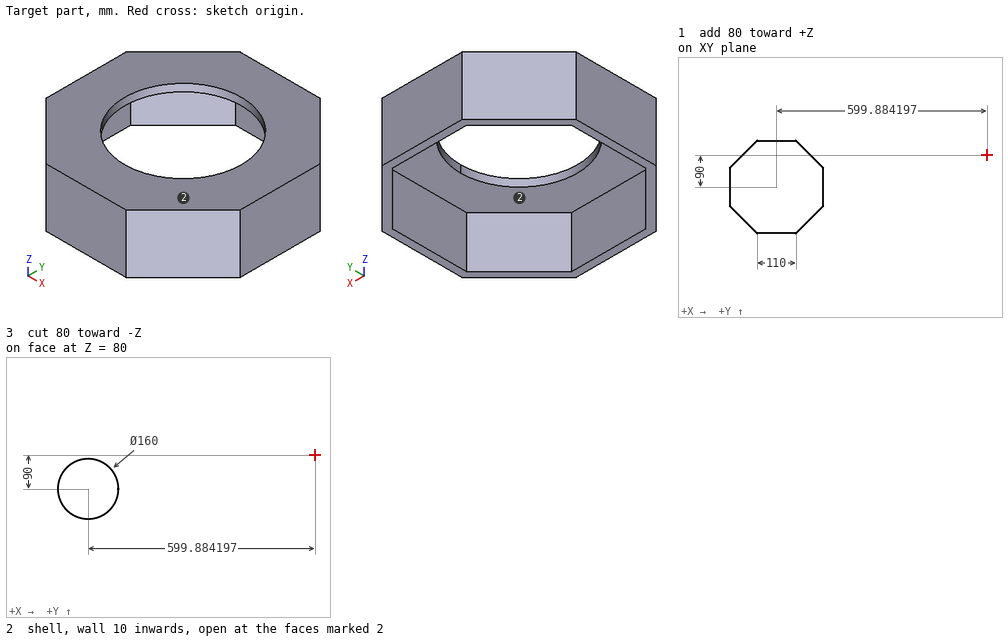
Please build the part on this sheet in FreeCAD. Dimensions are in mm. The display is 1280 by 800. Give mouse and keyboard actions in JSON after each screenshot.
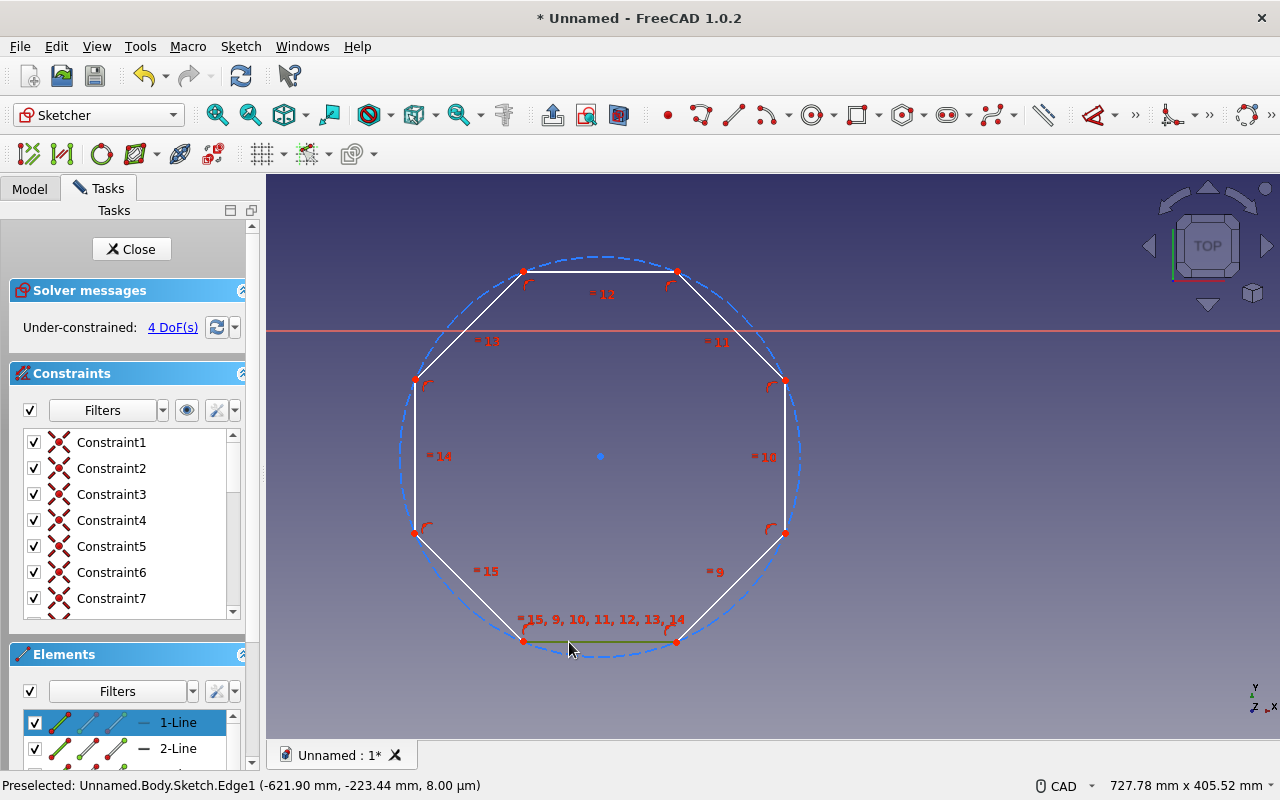
{"action": "key", "text": "h"}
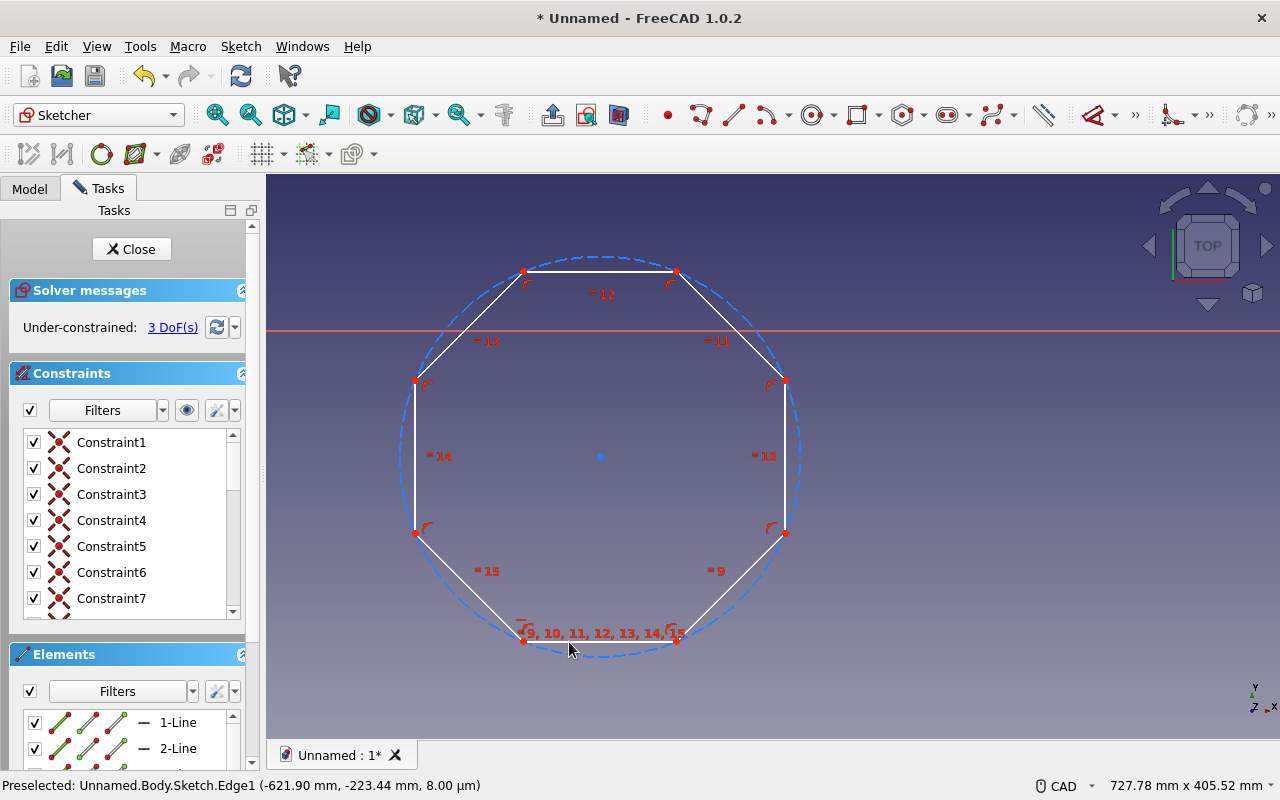
{"action": "left_click", "coordinate": [600, 457]}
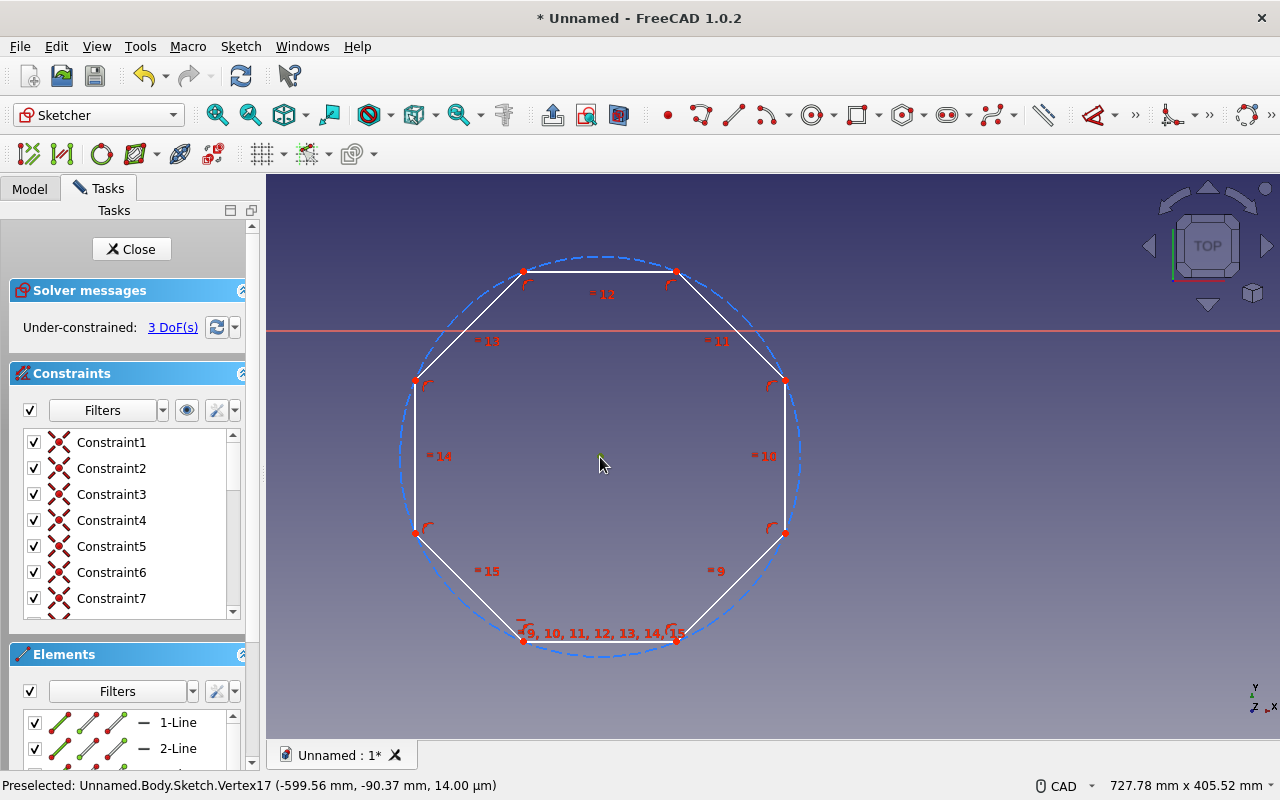
{"action": "key", "text": "i"}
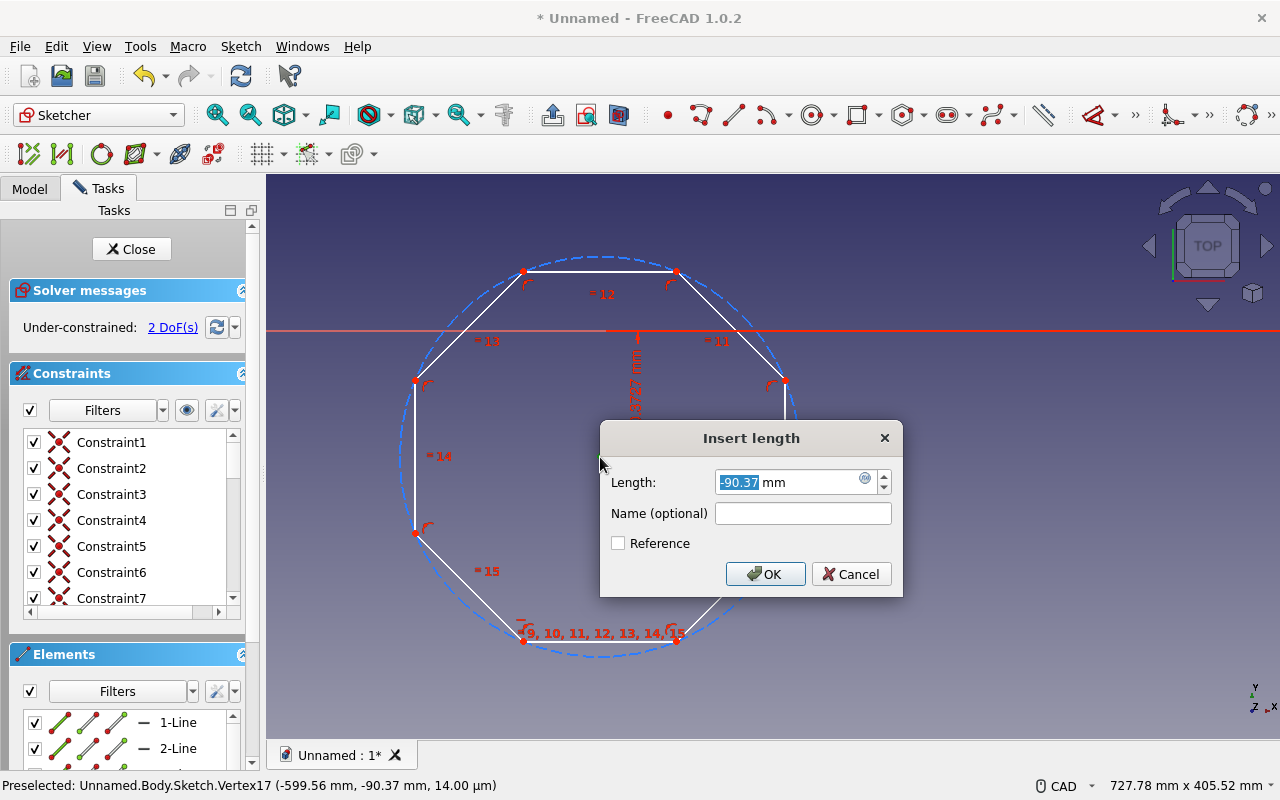
{"action": "type", "text": "-90"}
{"action": "key", "text": "Return"}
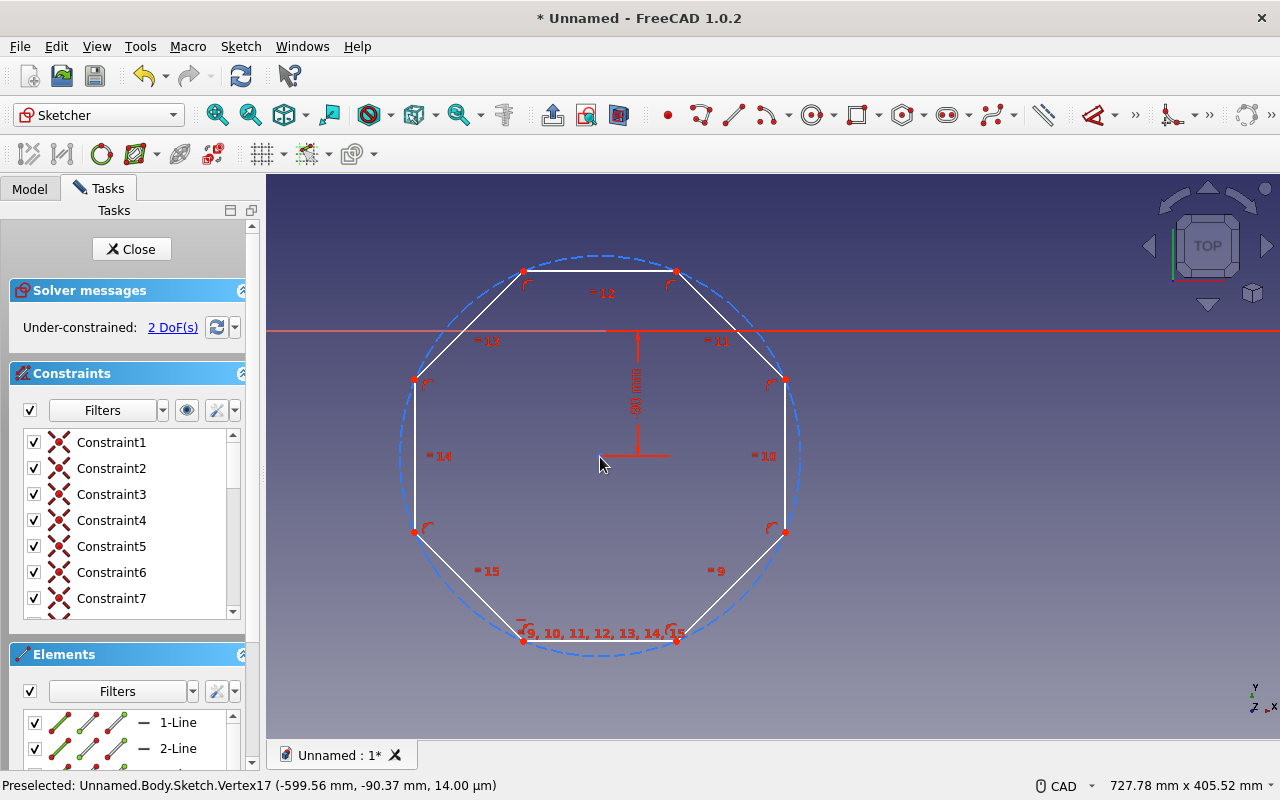
{"action": "left_click", "coordinate": [569, 641]}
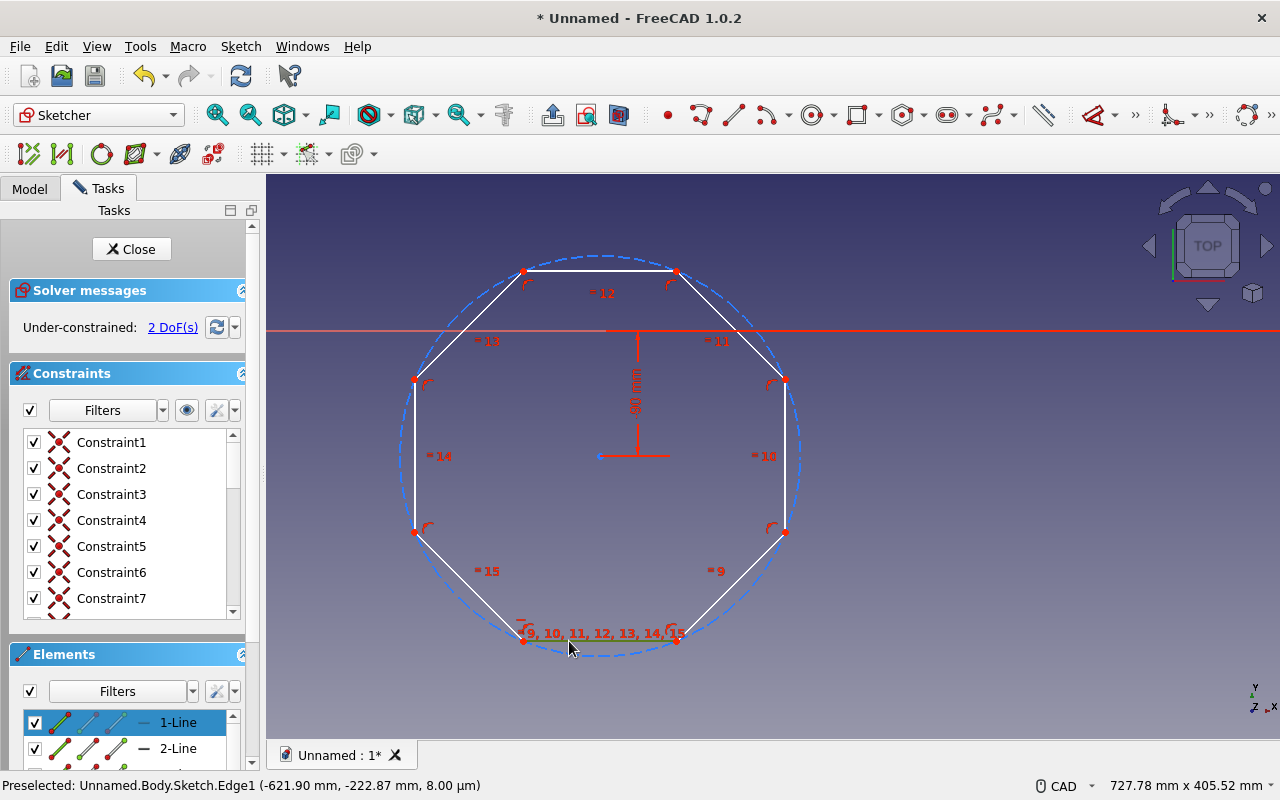
{"action": "key", "text": "l"}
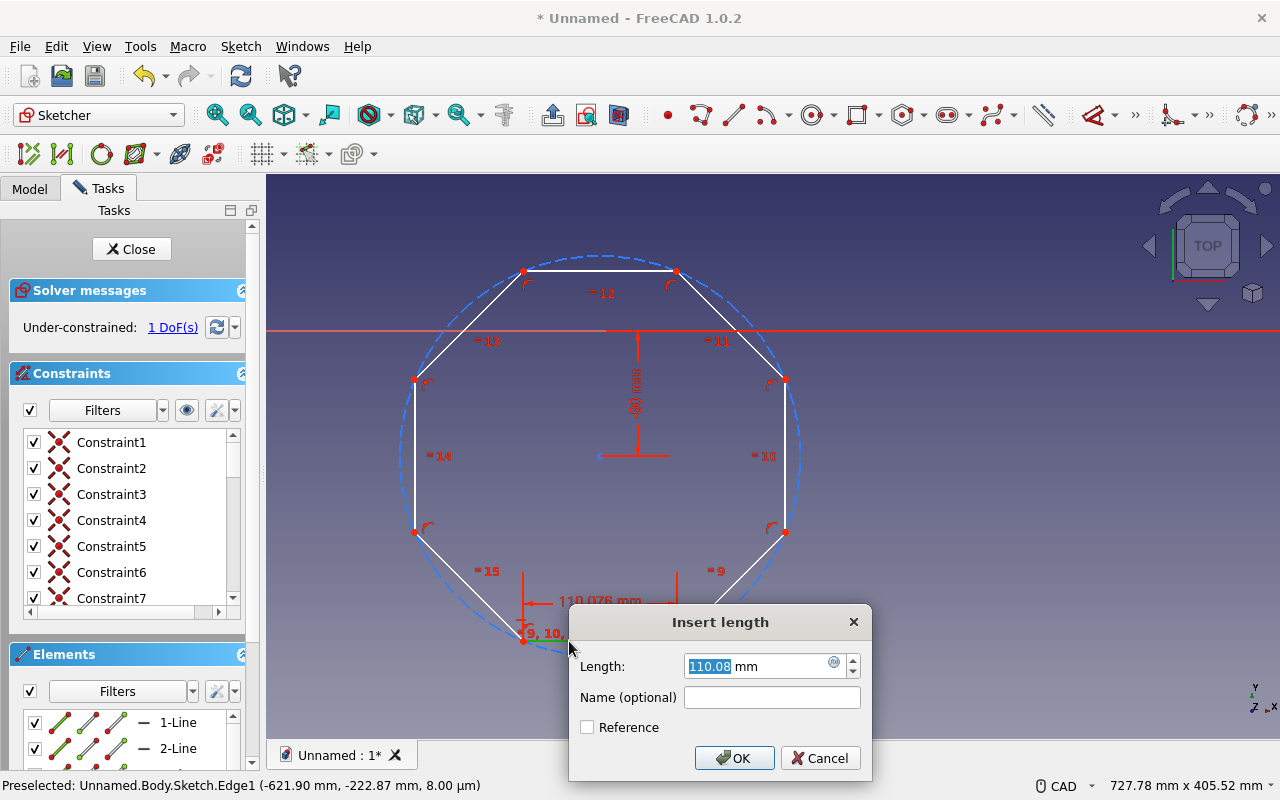
{"action": "type", "text": "110"}
{"action": "key", "text": "Return"}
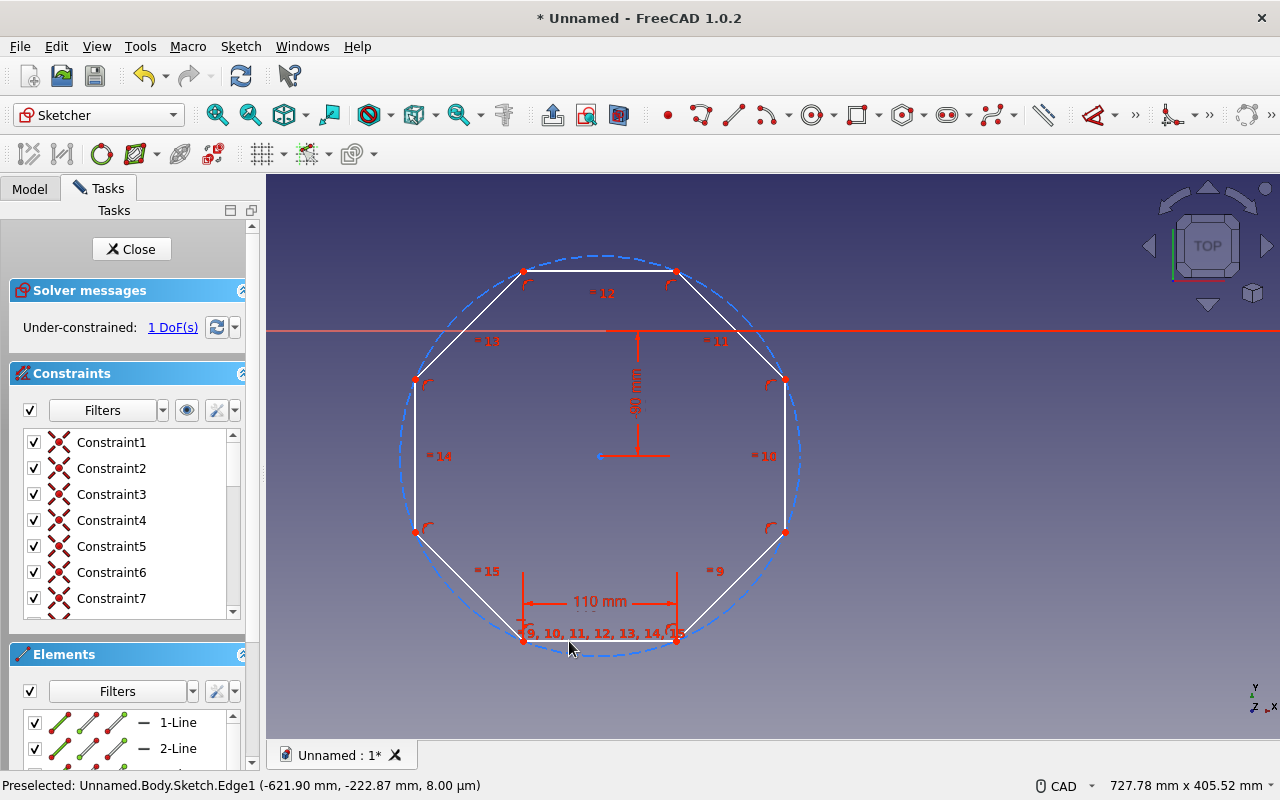
{"action": "left_click", "coordinate": [600, 456]}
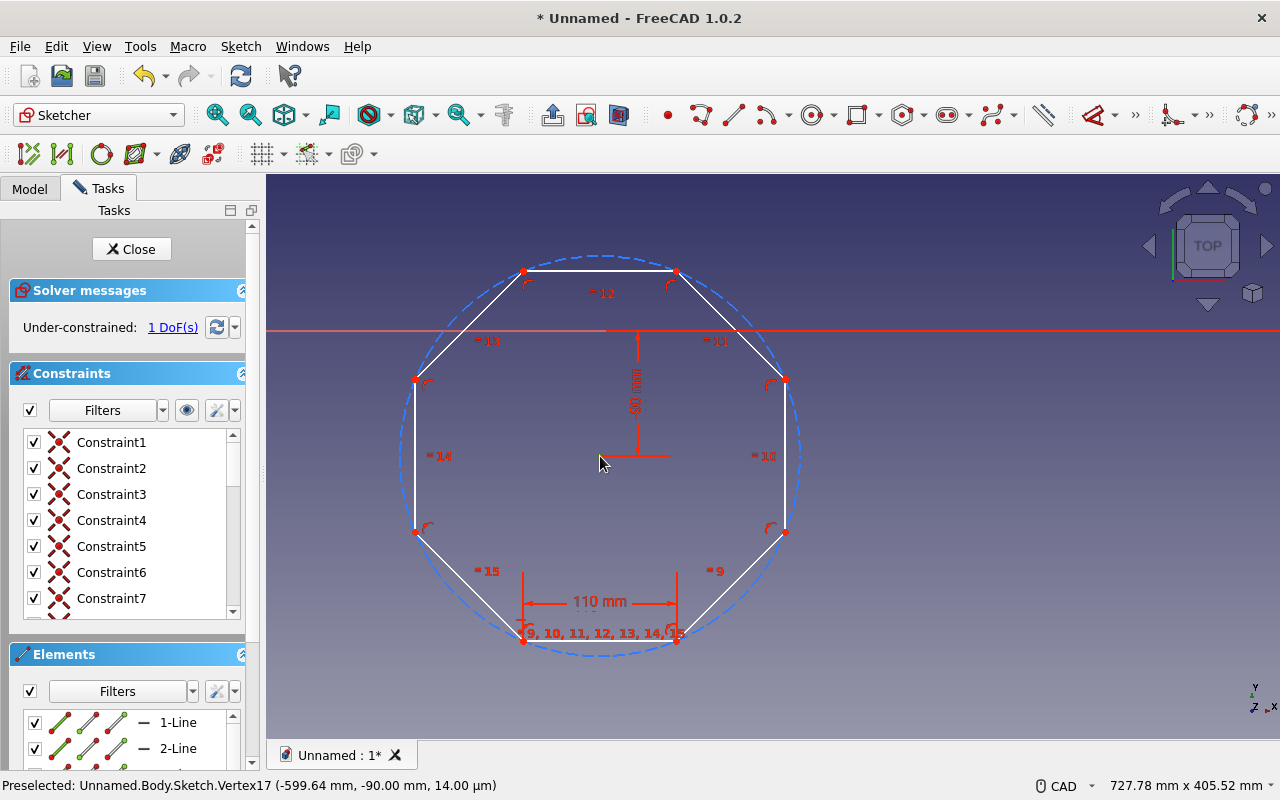
{"action": "key", "text": "l"}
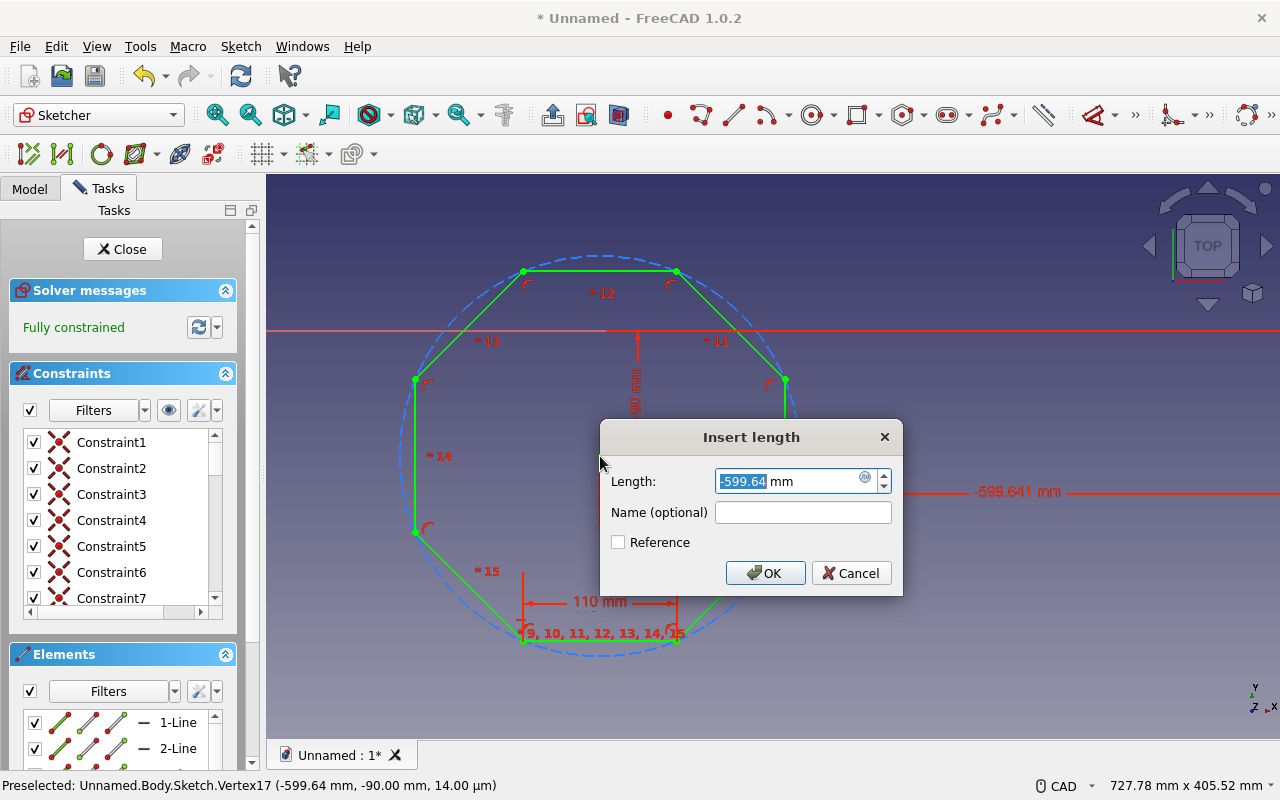
{"action": "type", "text": "-599.884197"}
{"action": "key", "text": "Return"}